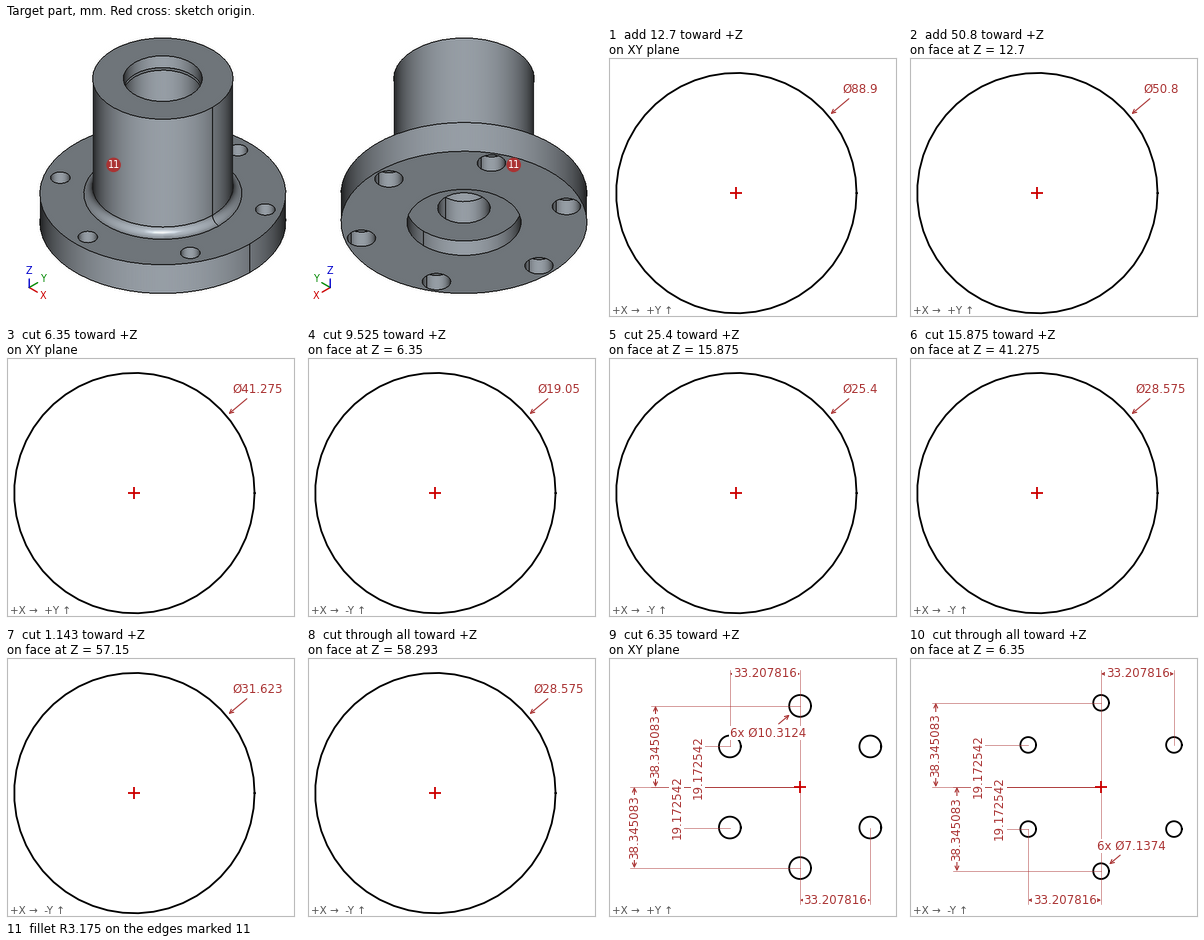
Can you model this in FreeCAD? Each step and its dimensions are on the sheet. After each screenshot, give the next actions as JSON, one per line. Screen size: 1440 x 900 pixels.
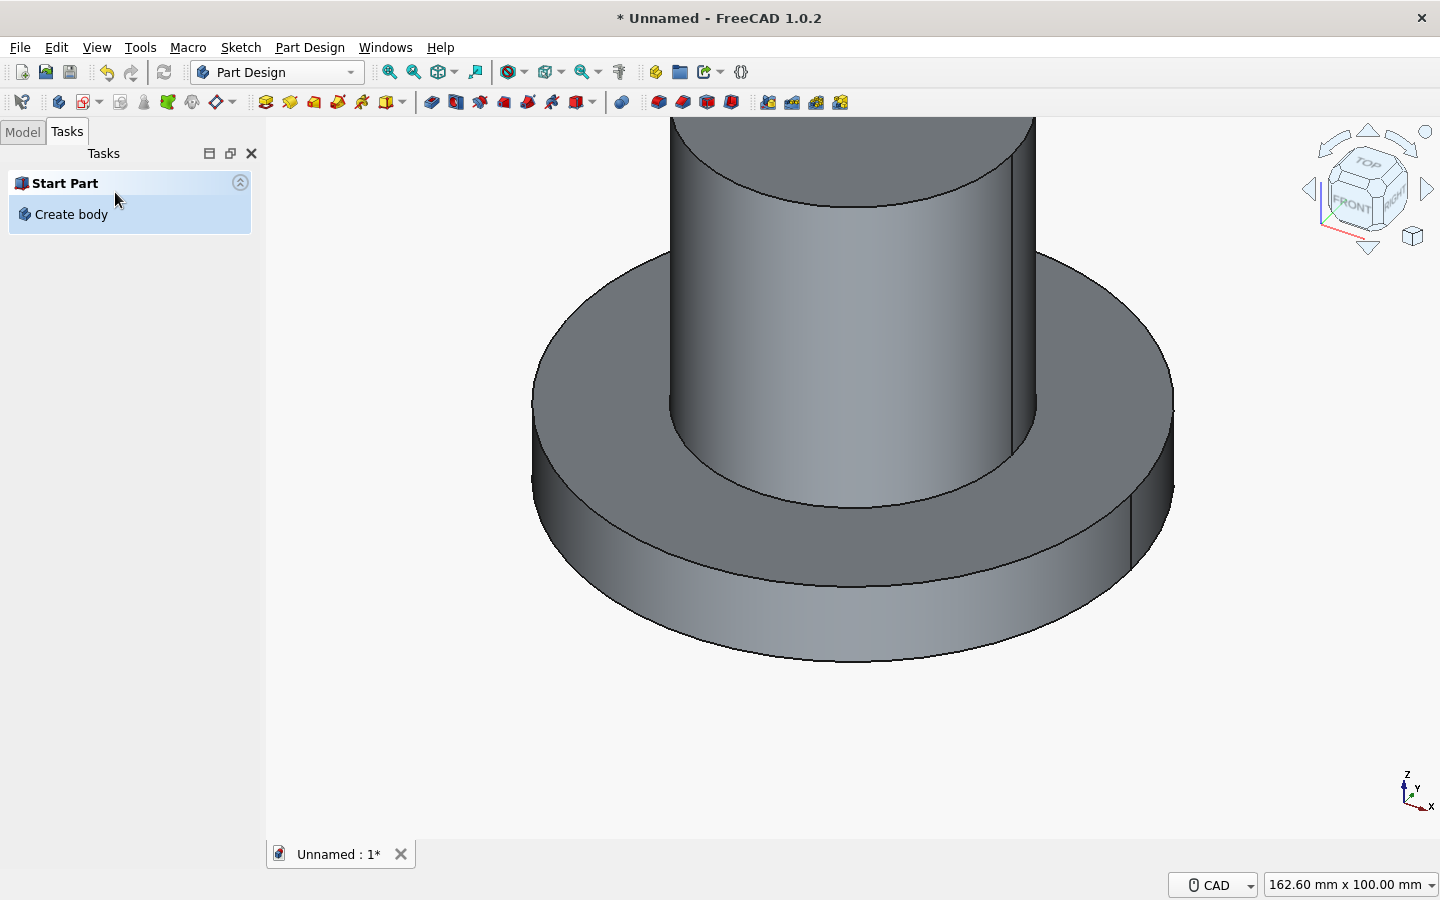
{"action": "left_click", "coordinate": [390, 72]}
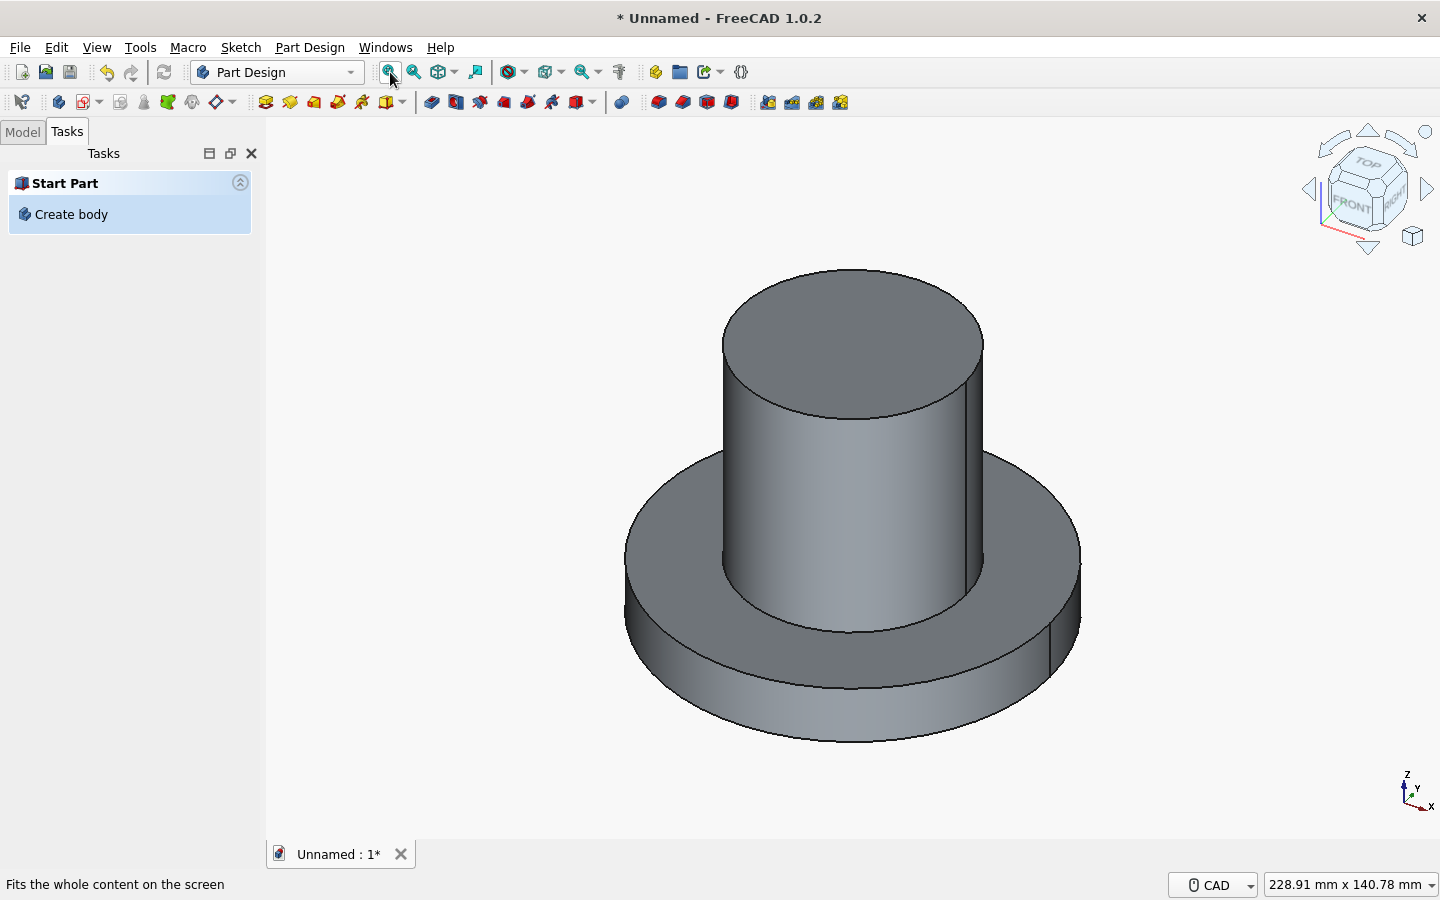
{"action": "left_click", "coordinate": [84, 102]}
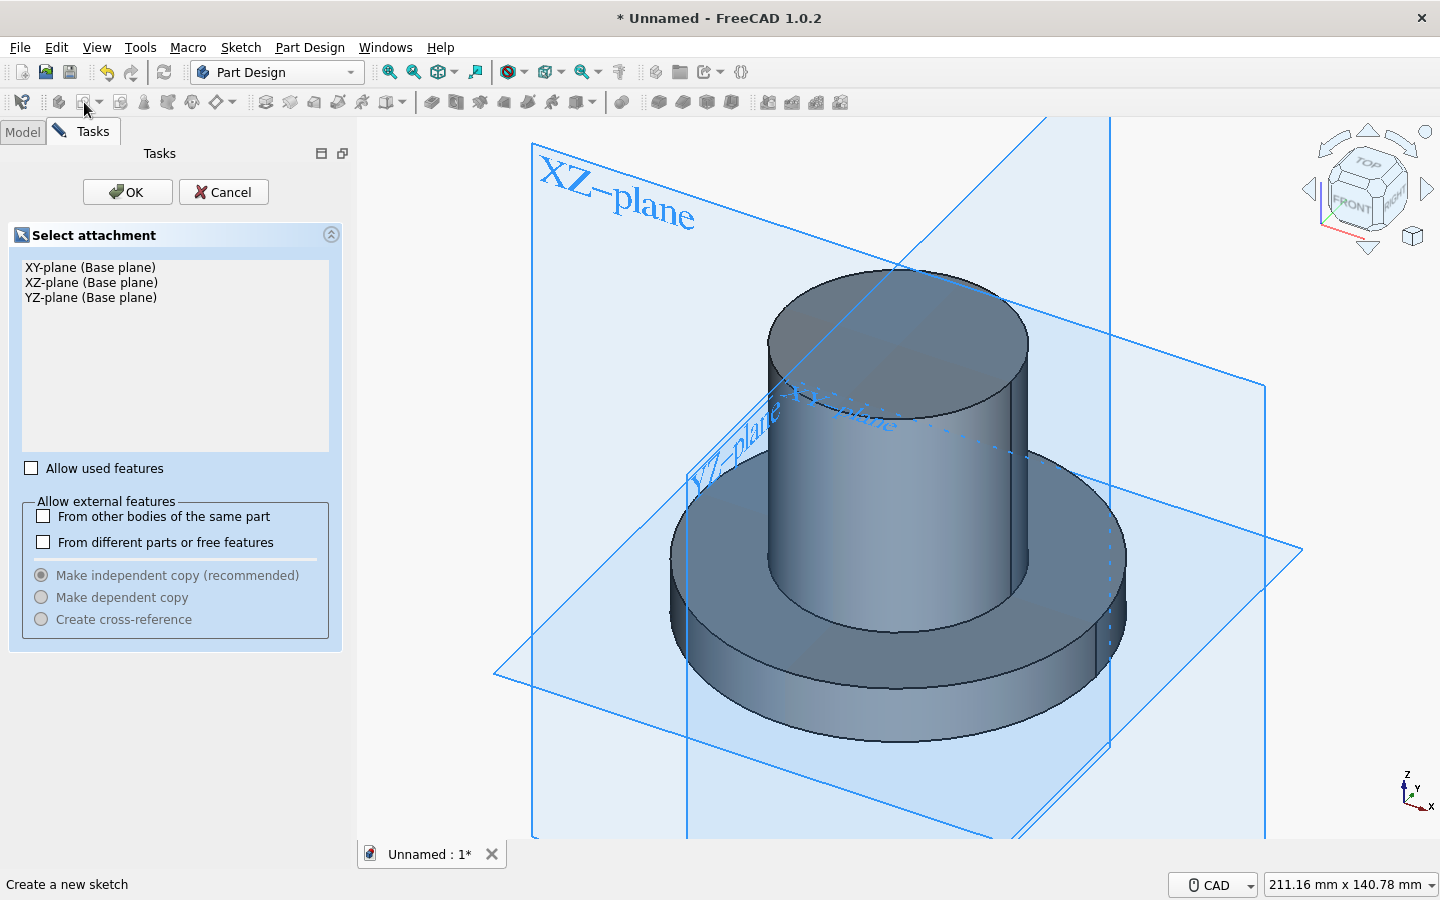
{"action": "left_click", "coordinate": [82, 268]}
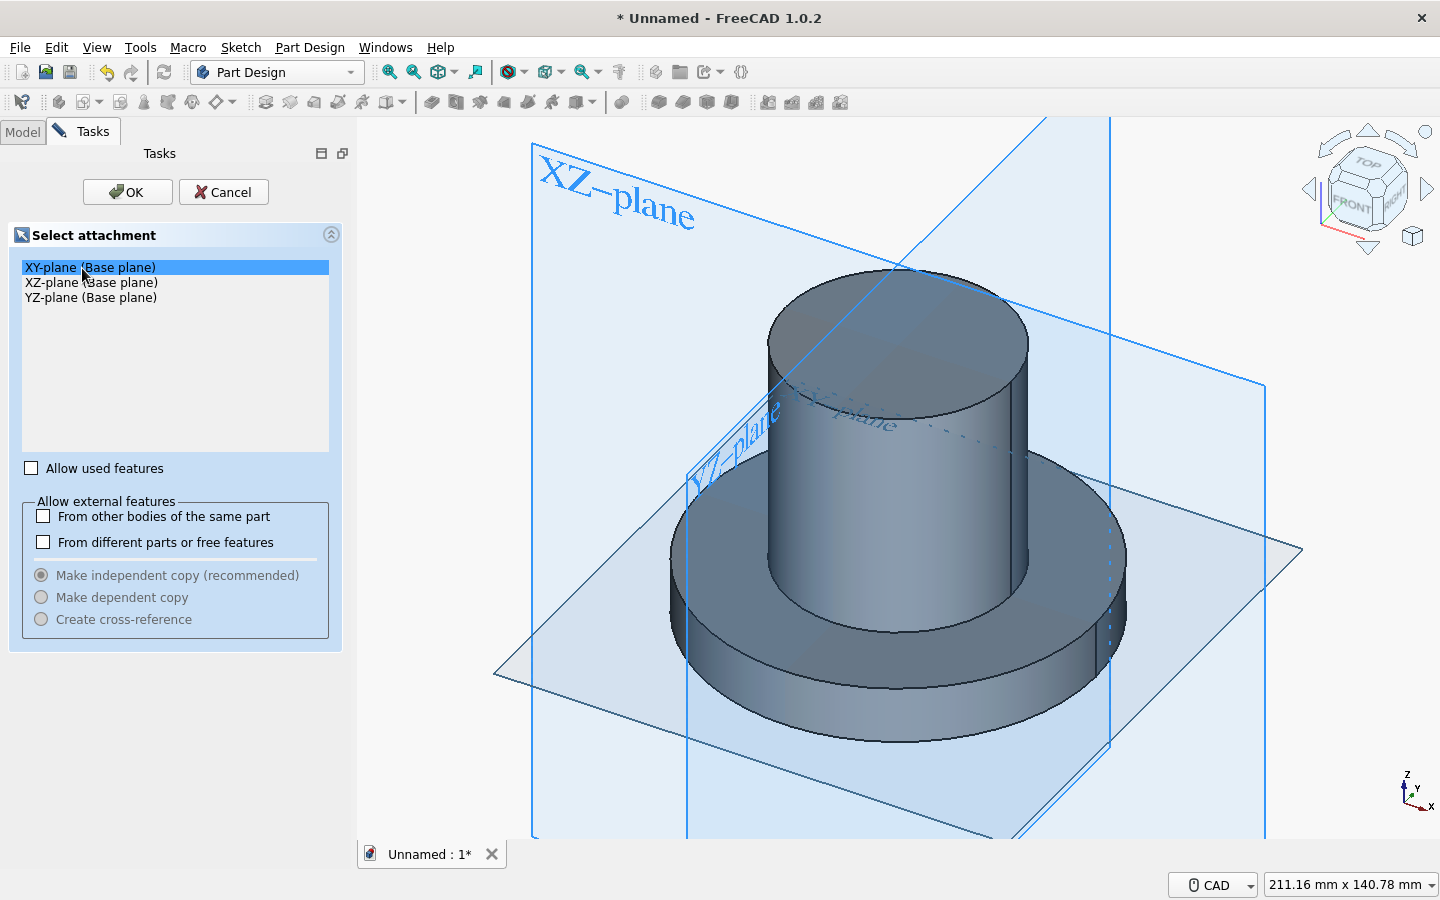
{"action": "left_click", "coordinate": [128, 192]}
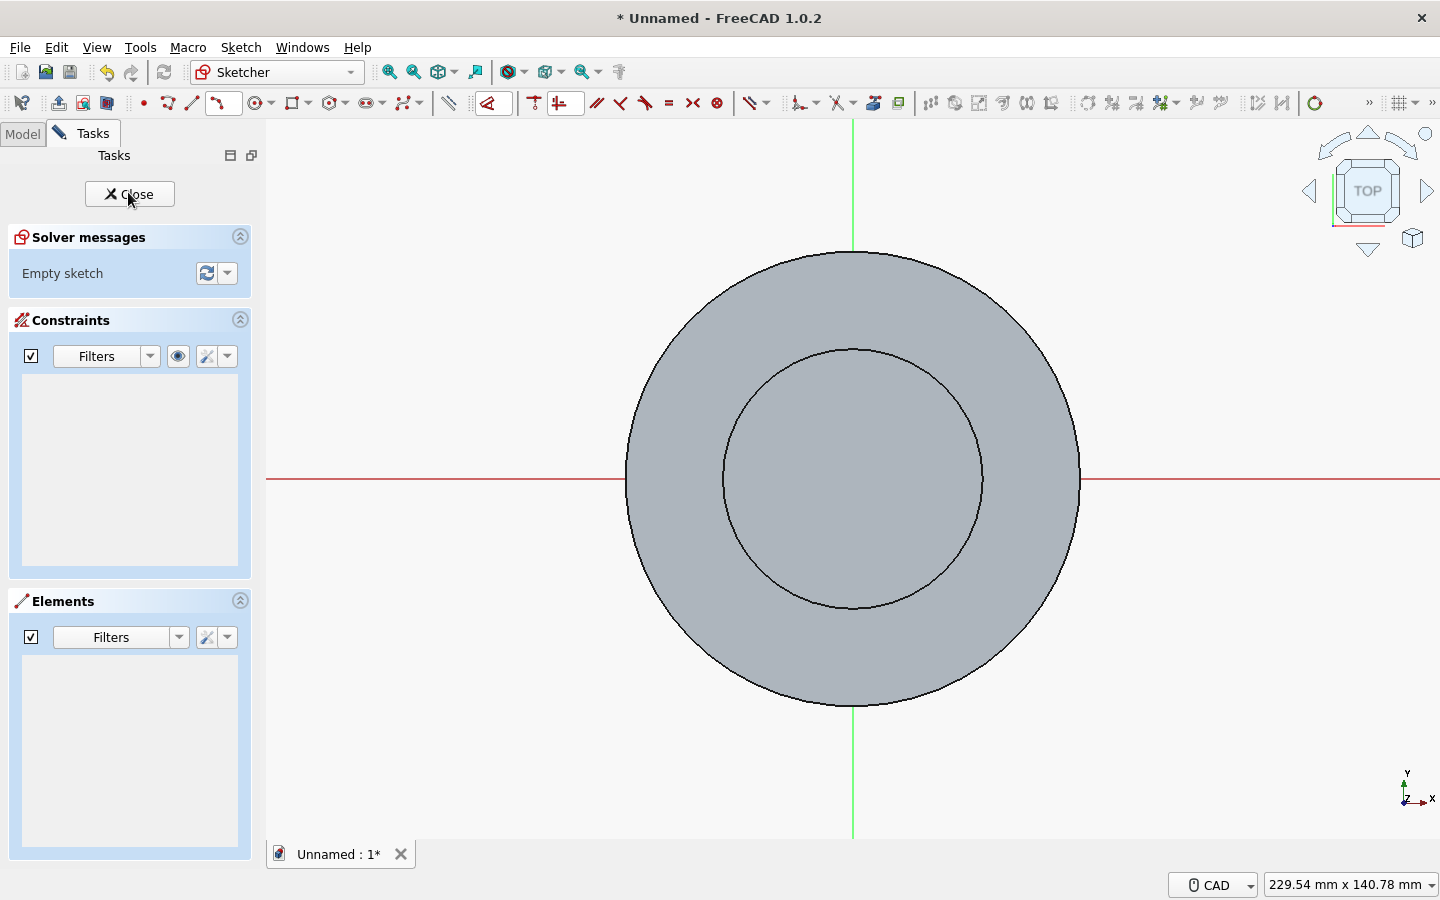
{"action": "key", "text": "q s"}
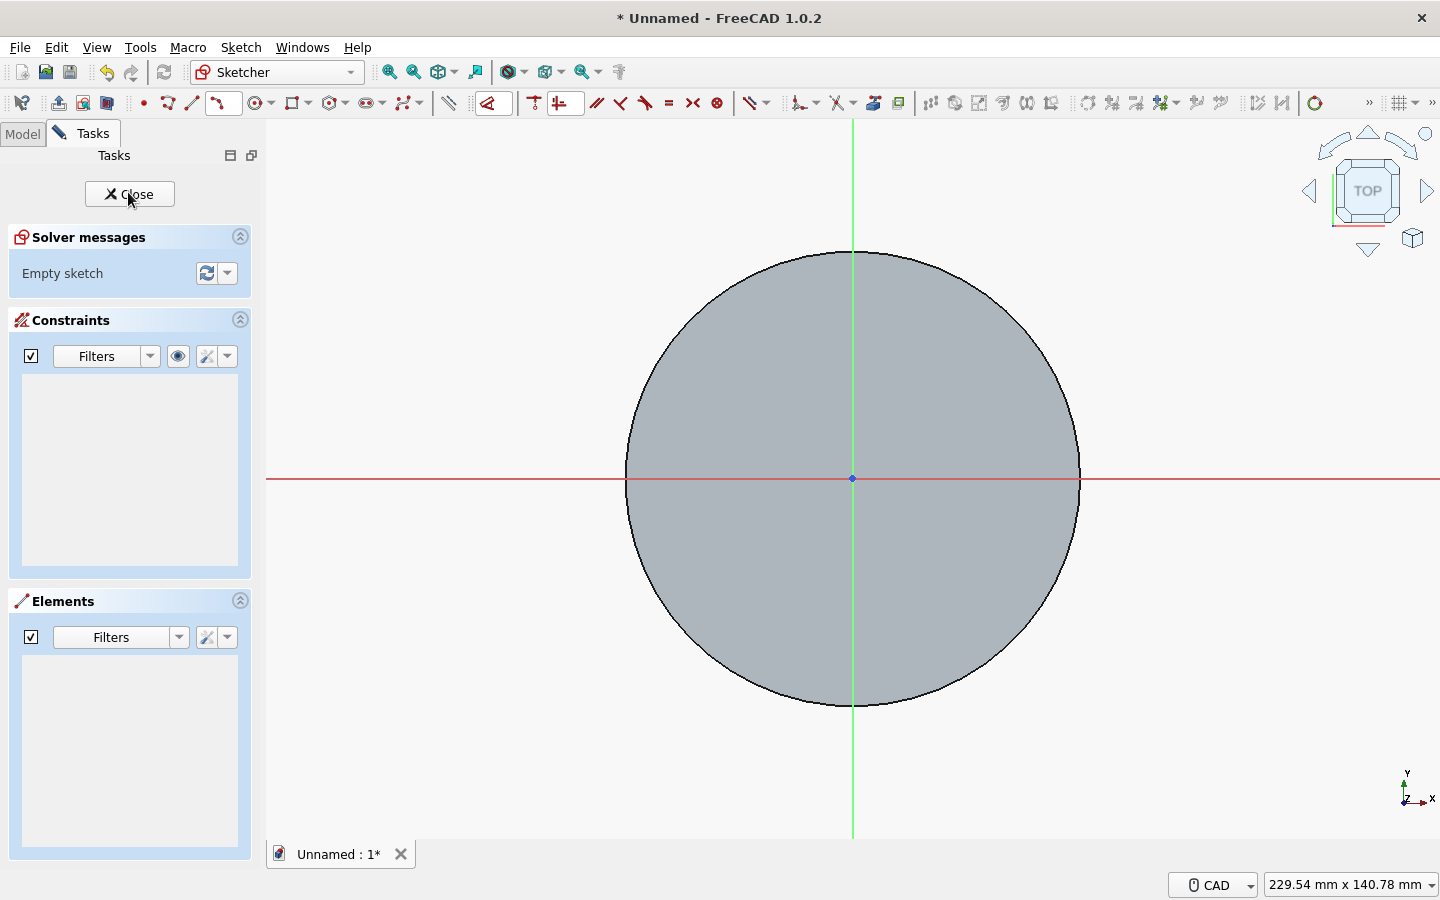
{"action": "scroll", "coordinate": [909, 479], "scroll_direction": "up", "scroll_amount": 4}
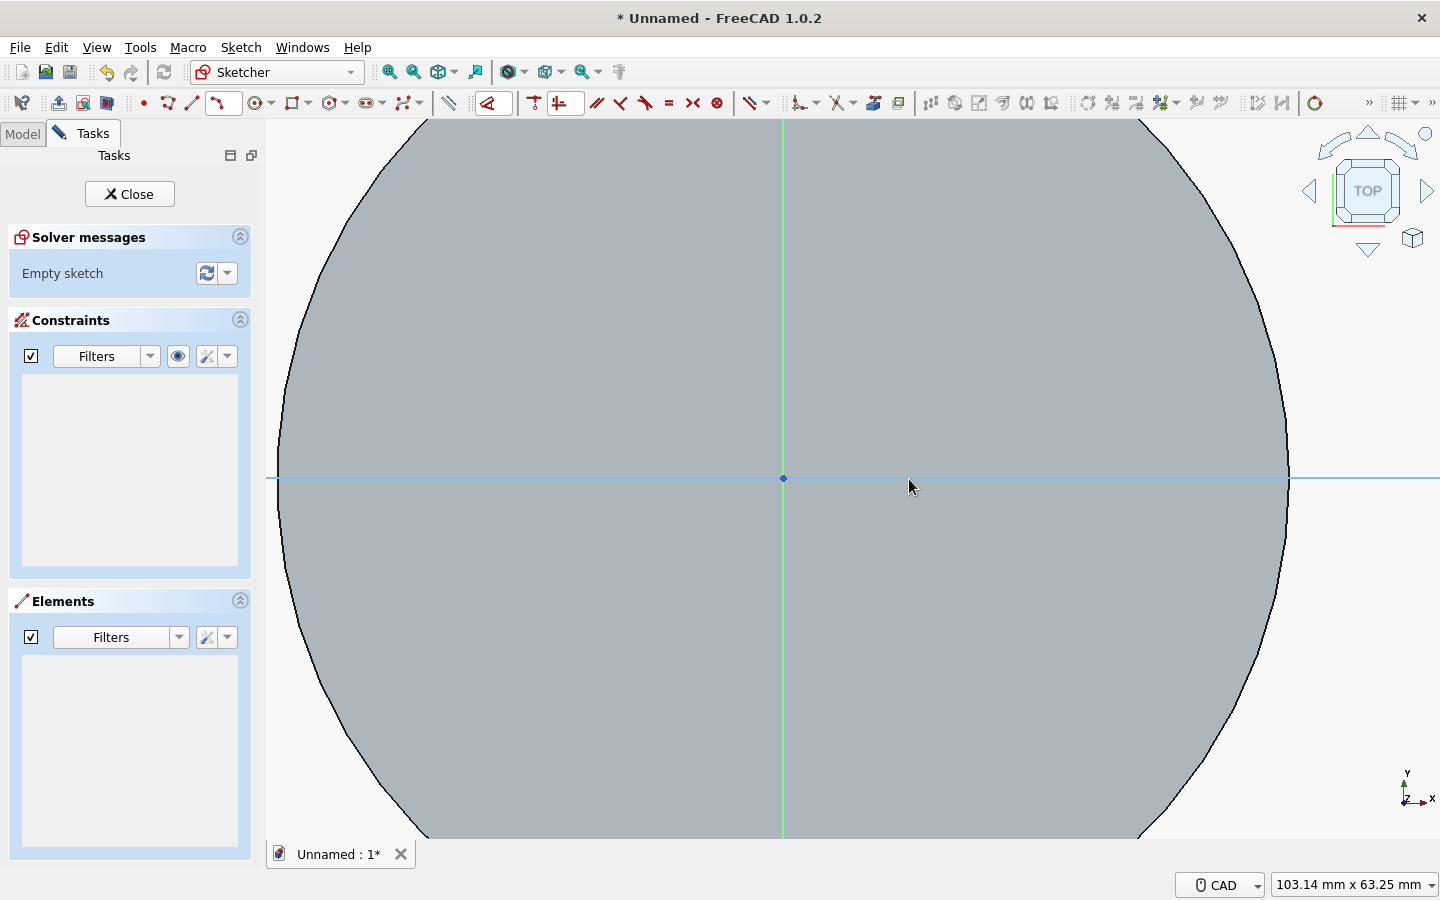
{"action": "left_click", "coordinate": [256, 104]}